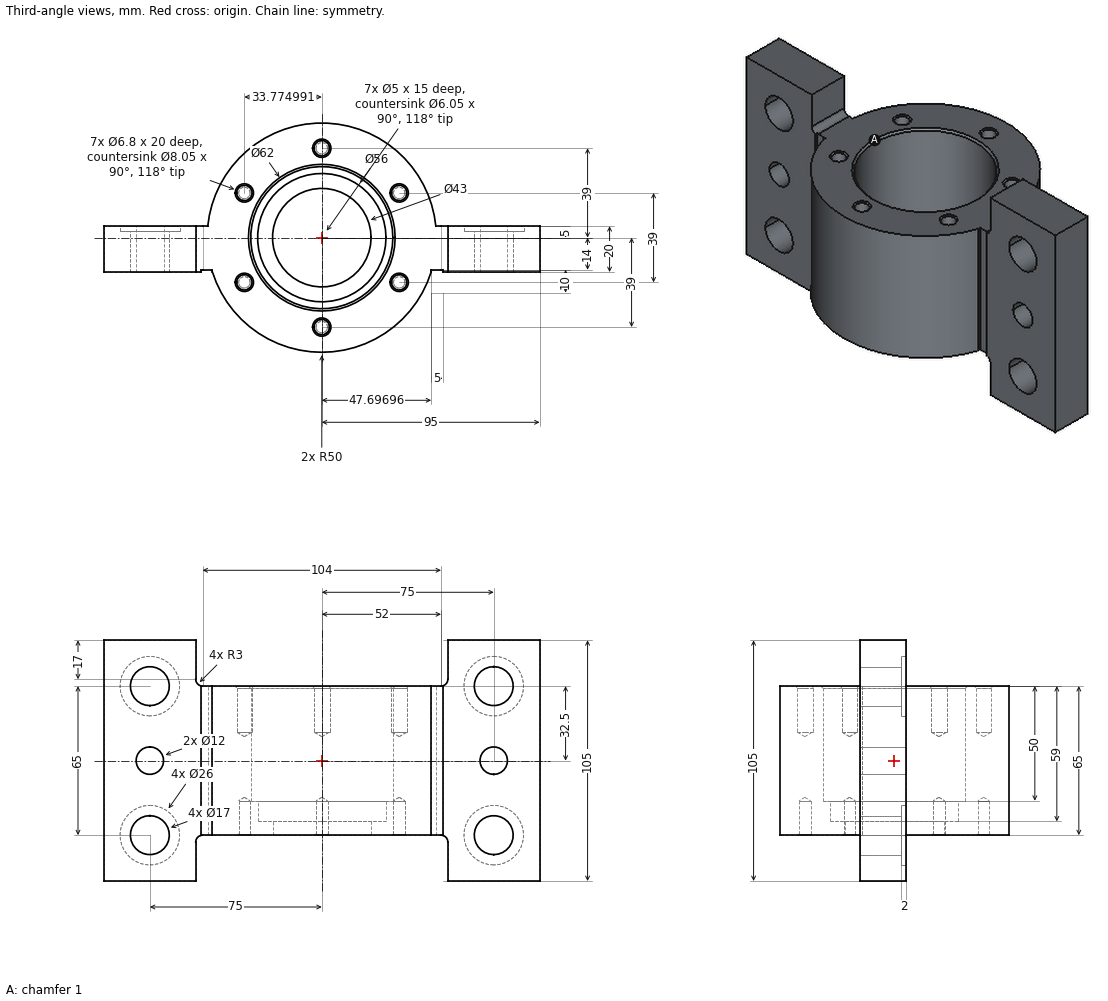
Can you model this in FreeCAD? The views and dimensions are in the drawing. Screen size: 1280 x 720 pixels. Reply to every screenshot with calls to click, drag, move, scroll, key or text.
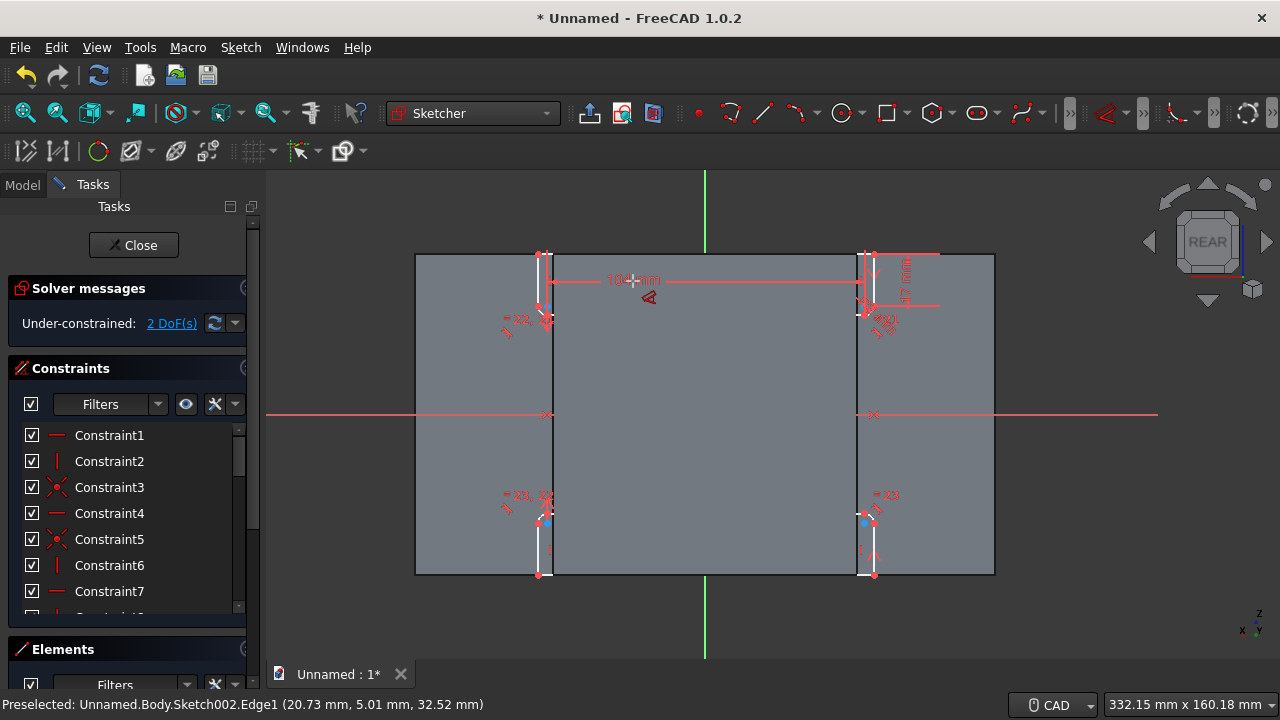
scroll(547, 315, up, 2)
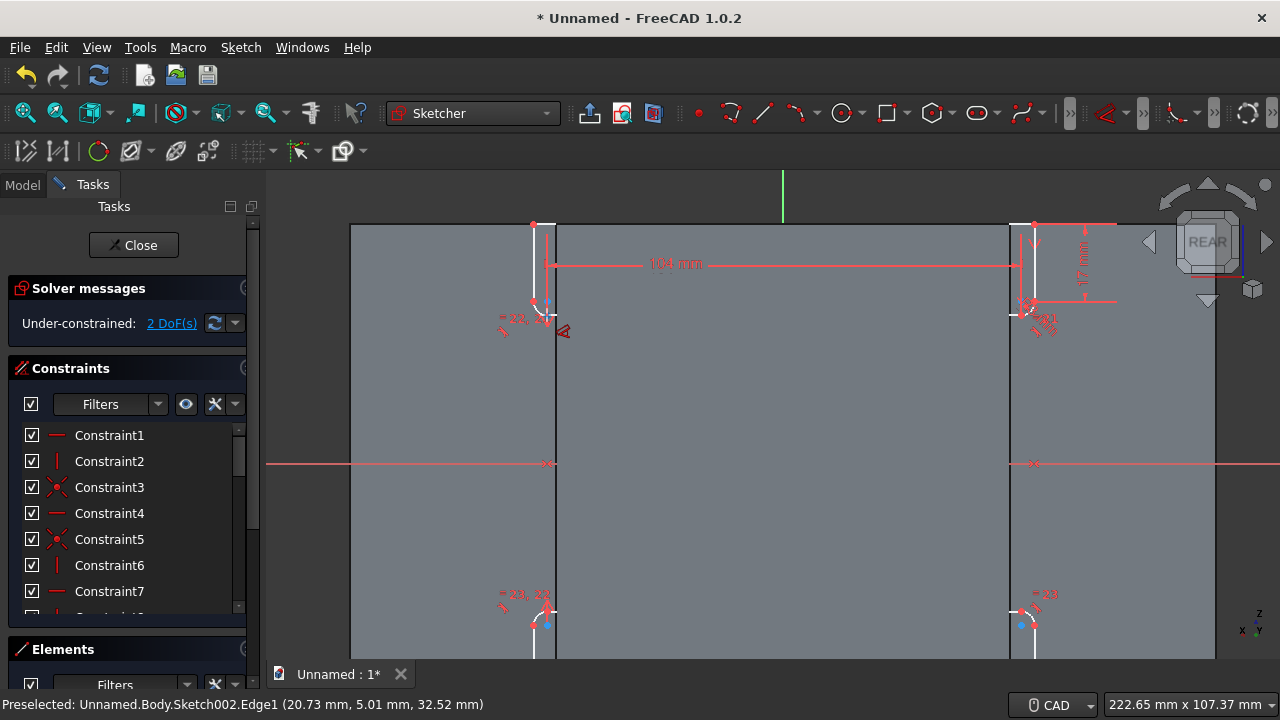
click(547, 315)
click(583, 281)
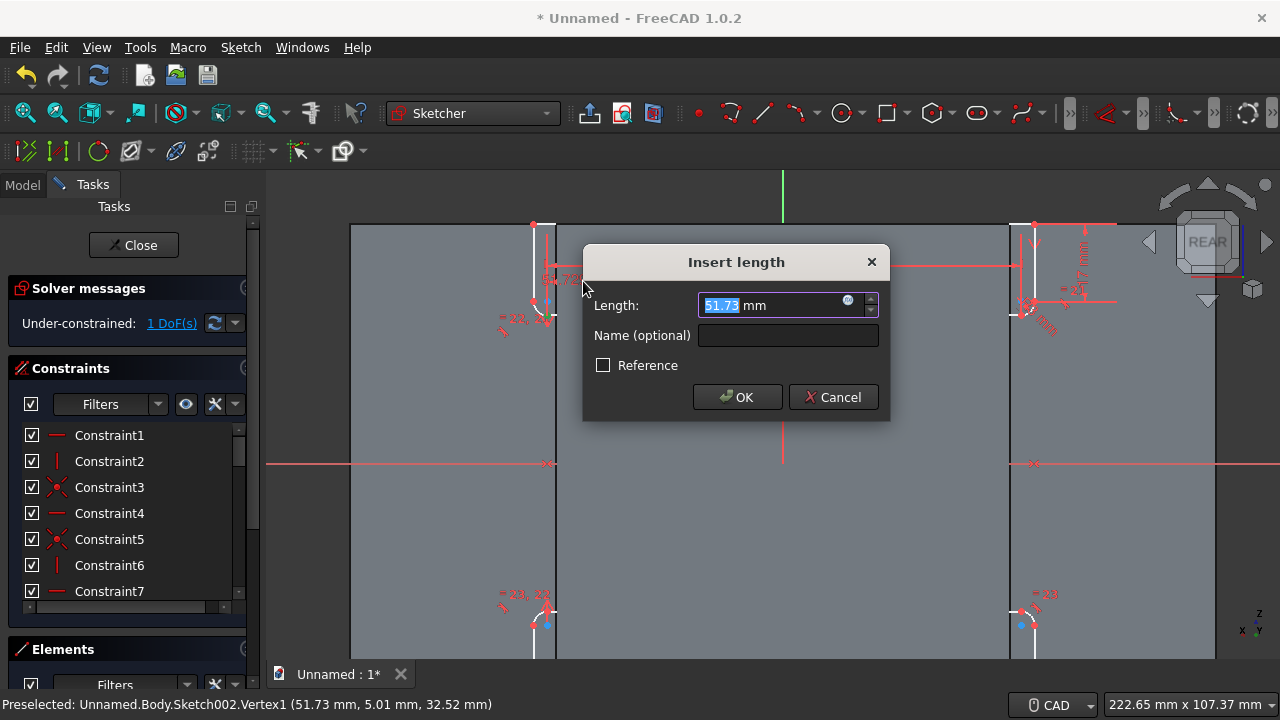
text(52)
key(Return)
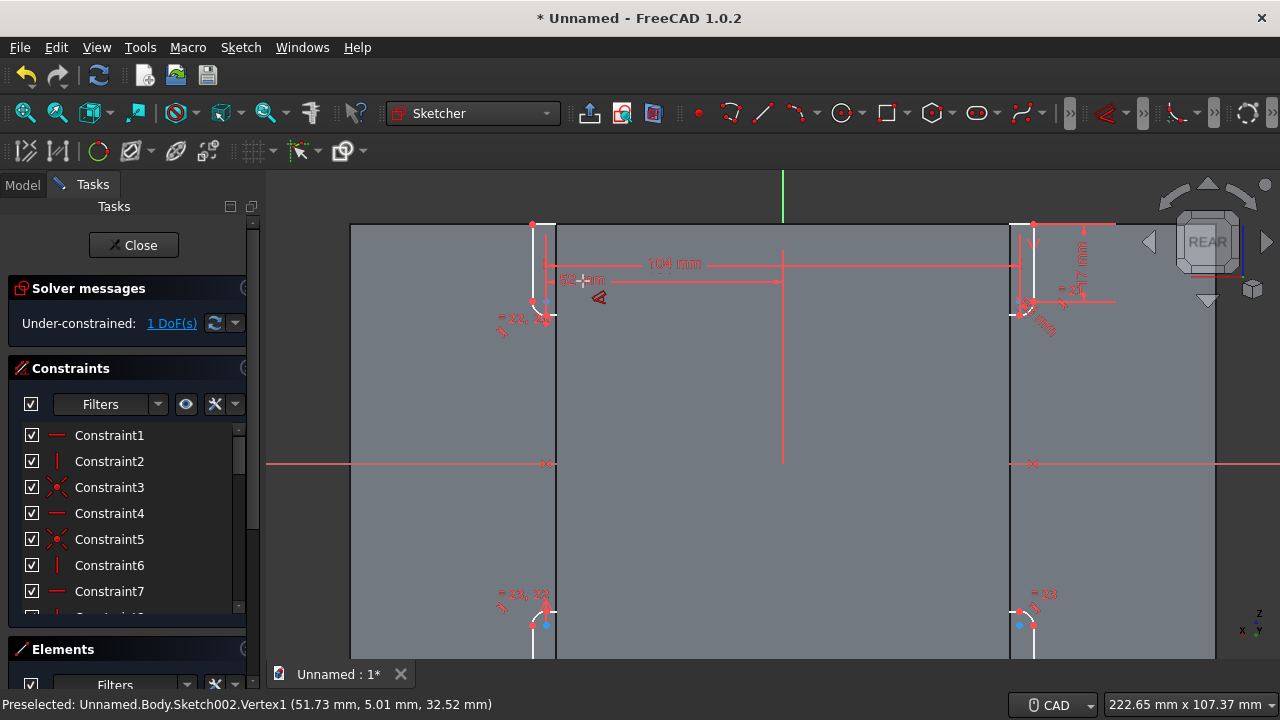
click(546, 315)
click(512, 390)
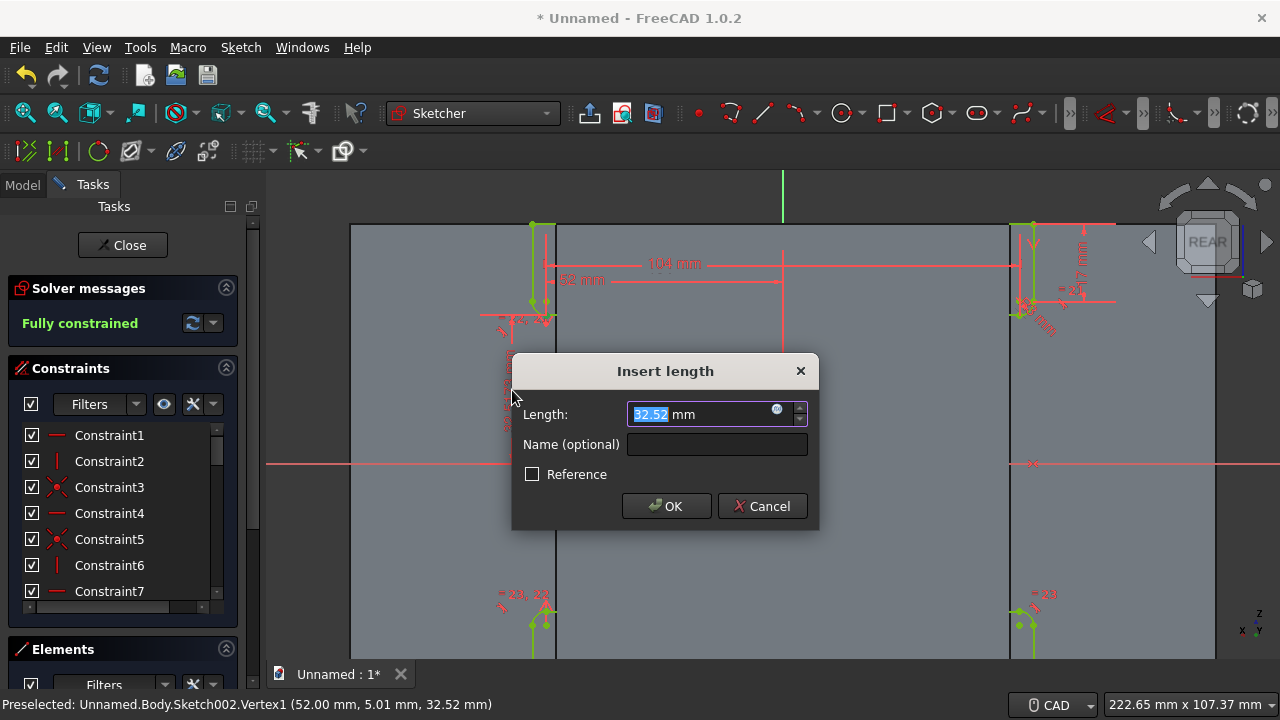
text(32.5)
key(Return)
key(Escape)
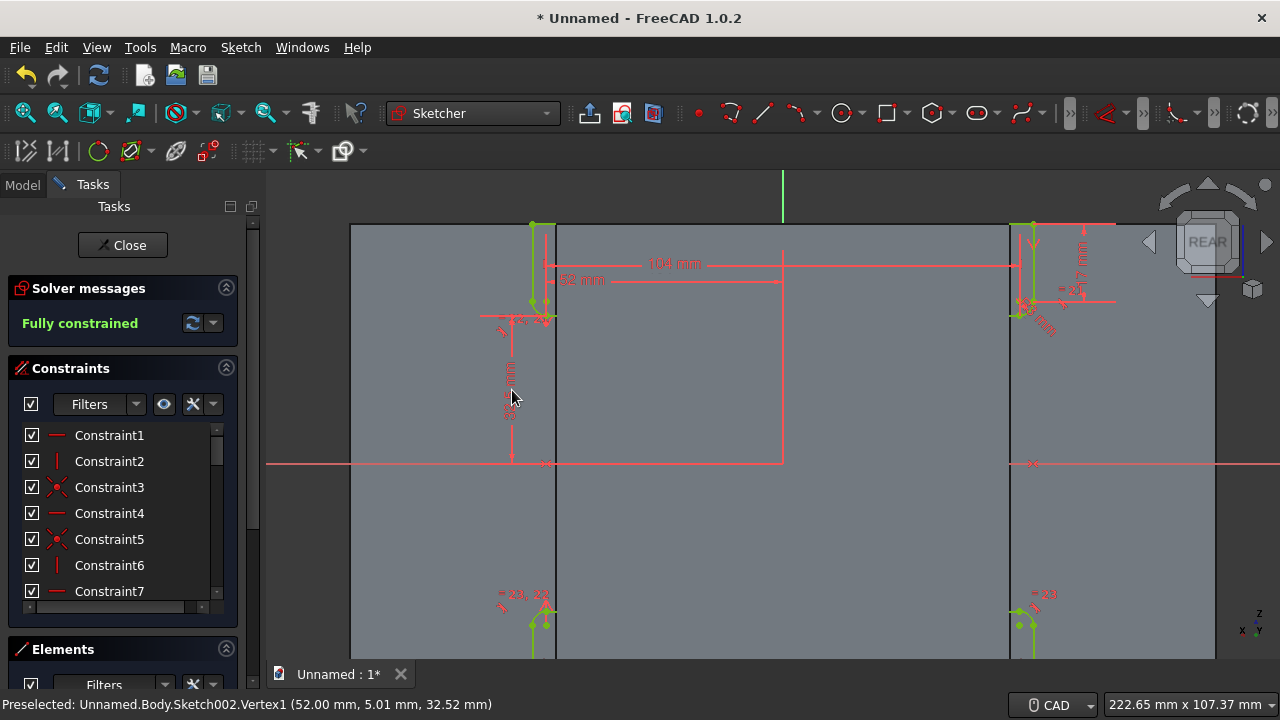
click(123, 245)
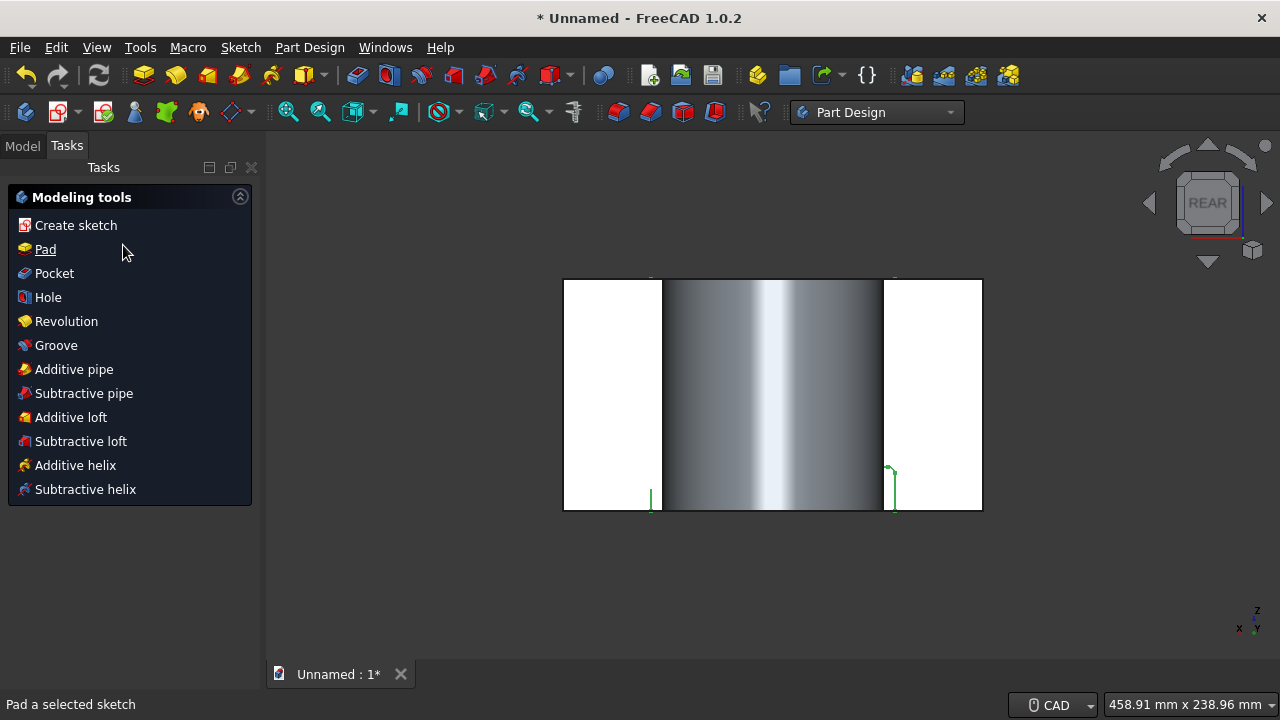
click(358, 76)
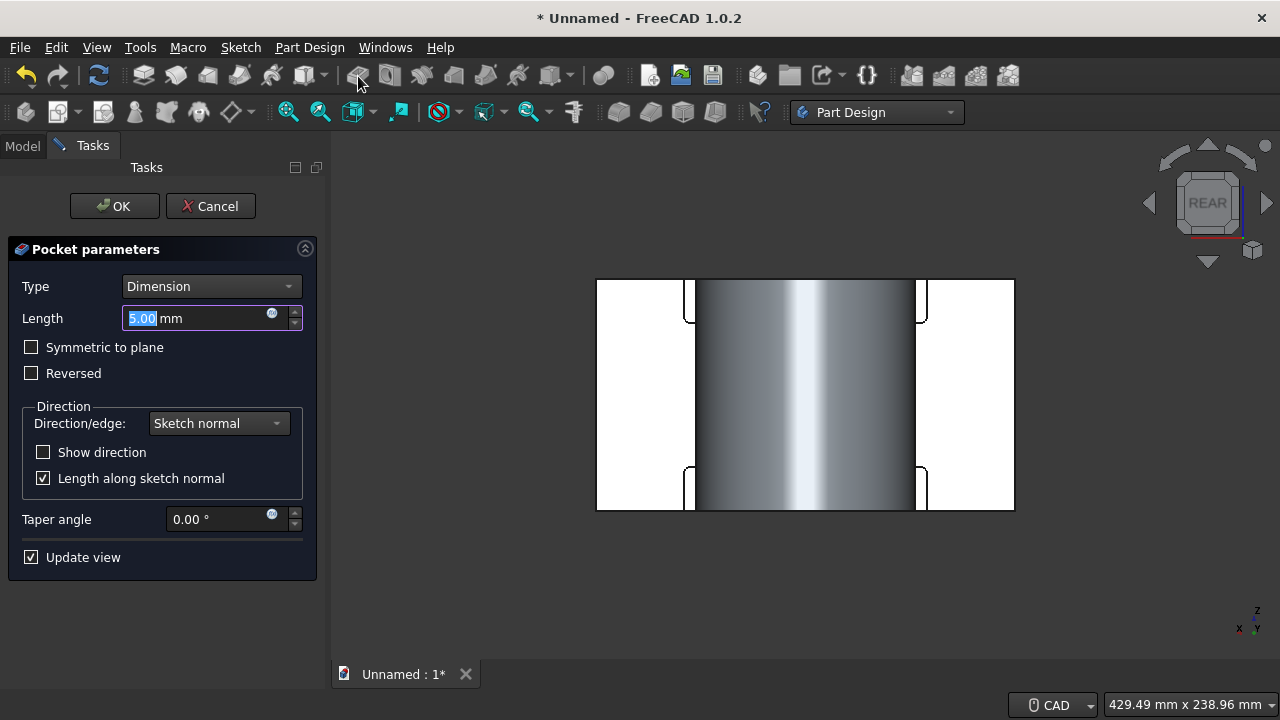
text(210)
key(Tab)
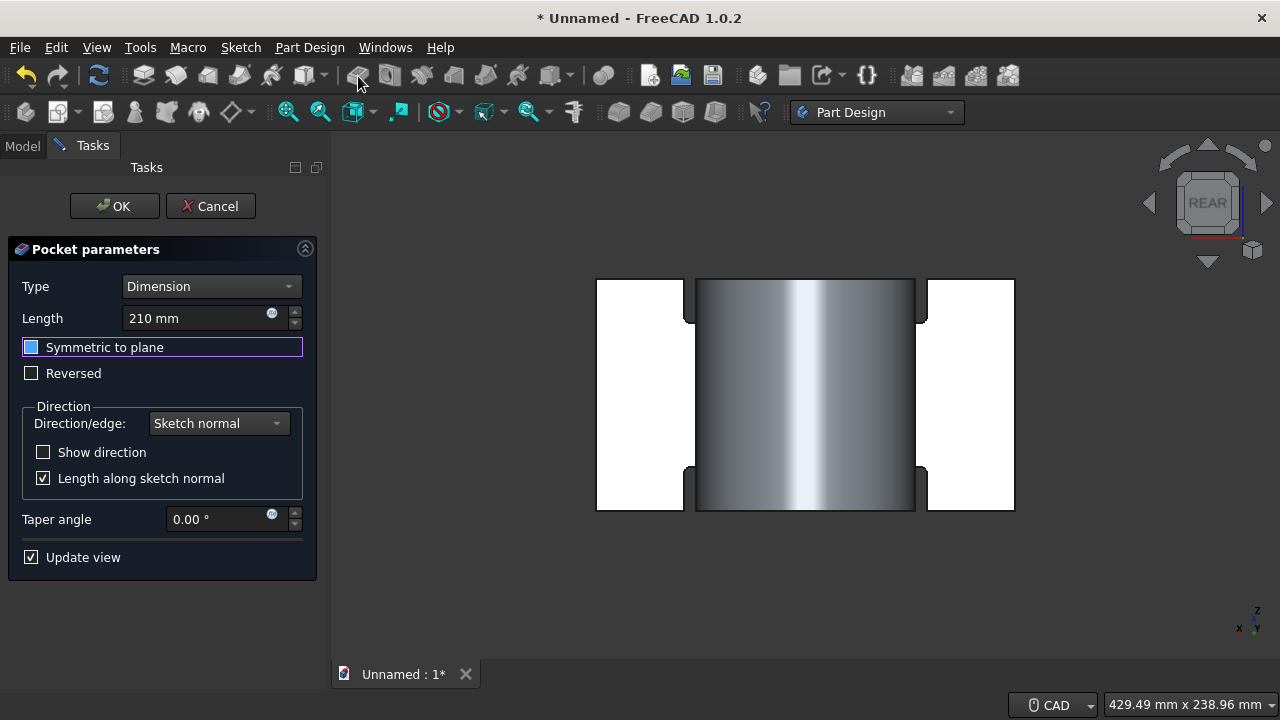
click(30, 347)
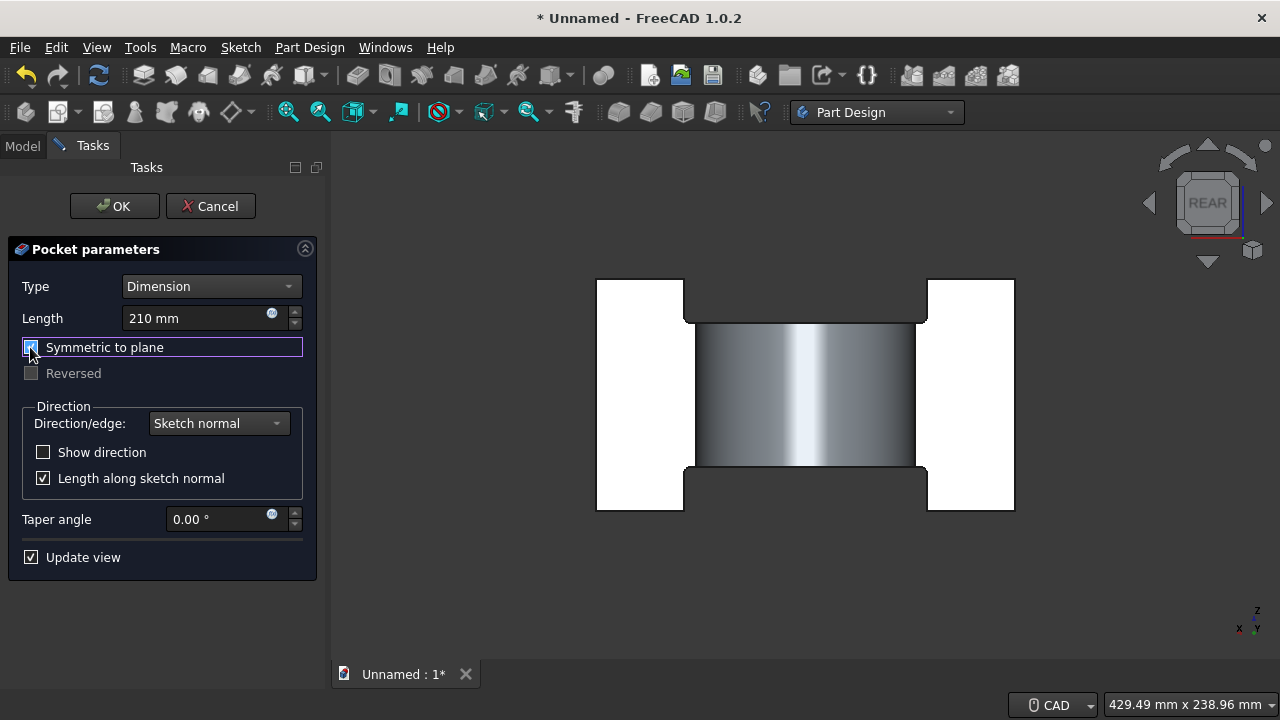
click(115, 206)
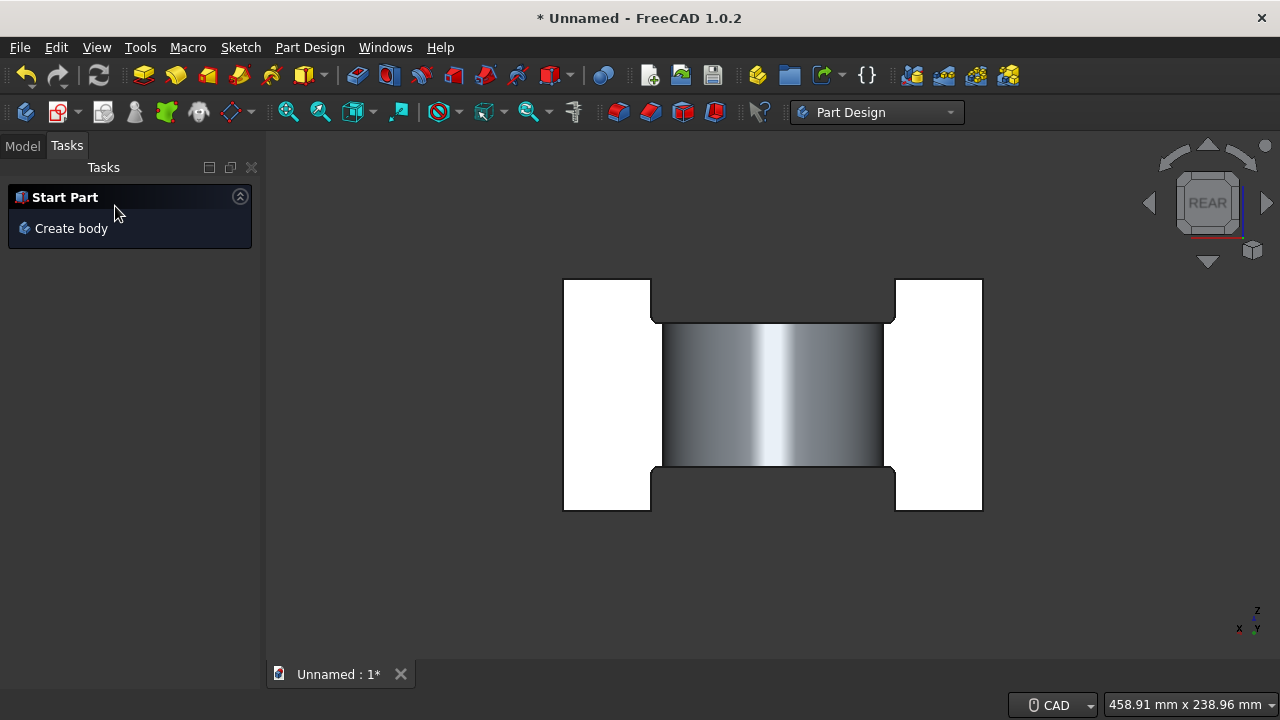
click(290, 112)